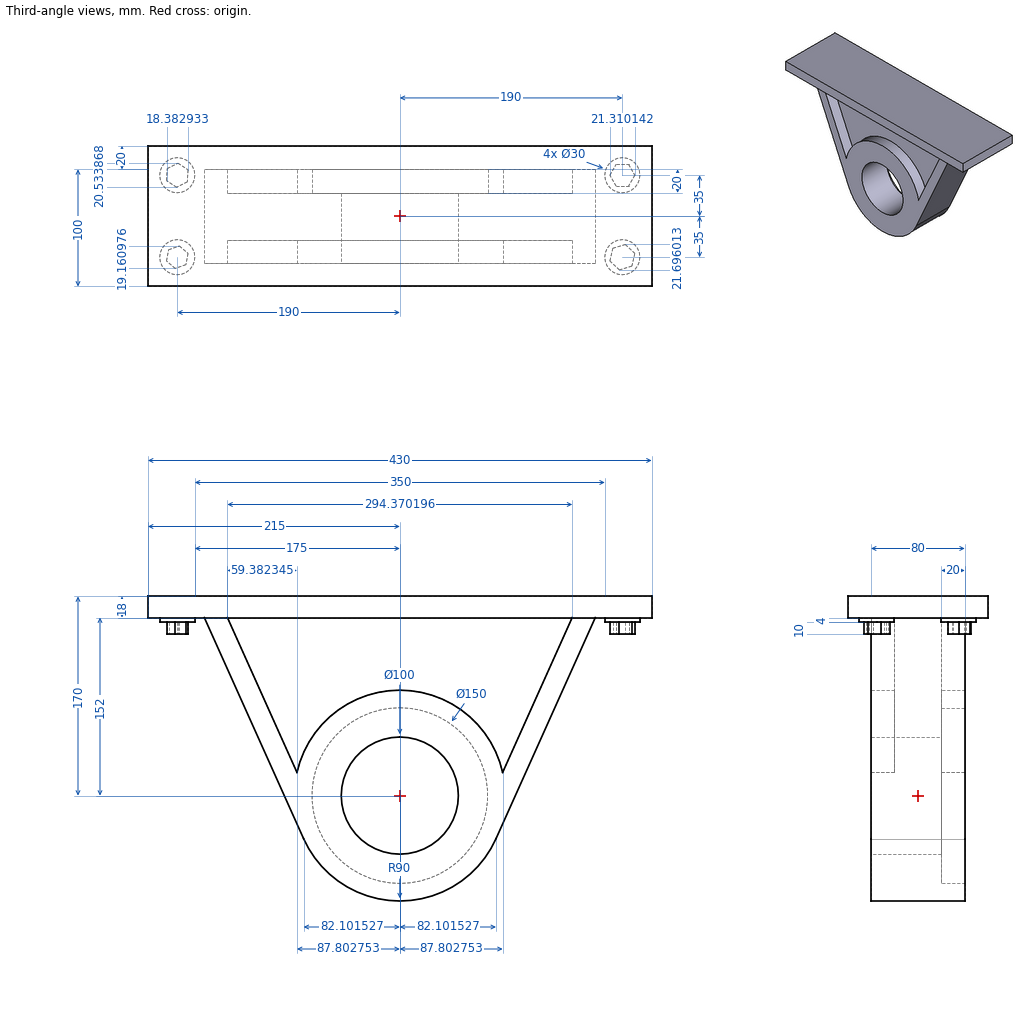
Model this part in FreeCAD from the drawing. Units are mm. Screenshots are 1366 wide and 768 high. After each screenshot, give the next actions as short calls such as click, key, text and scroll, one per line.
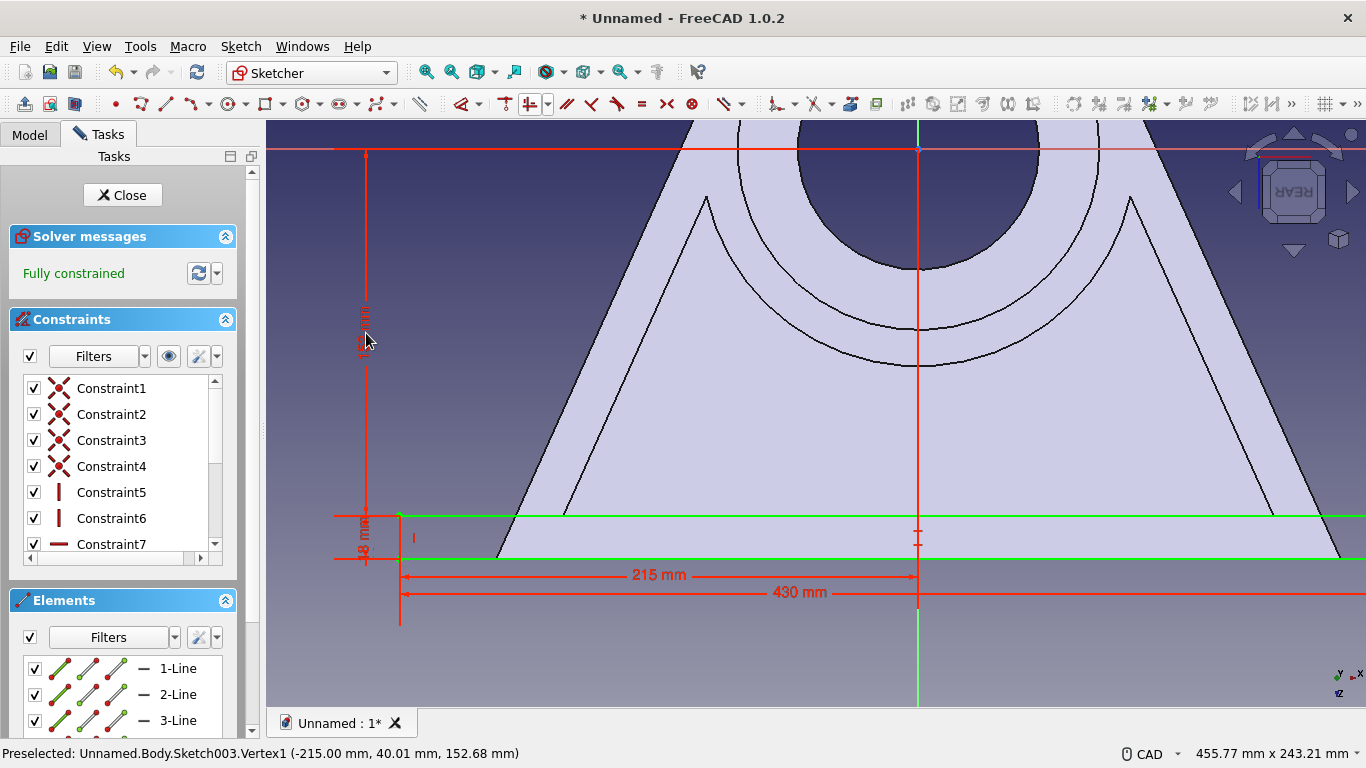
click(123, 195)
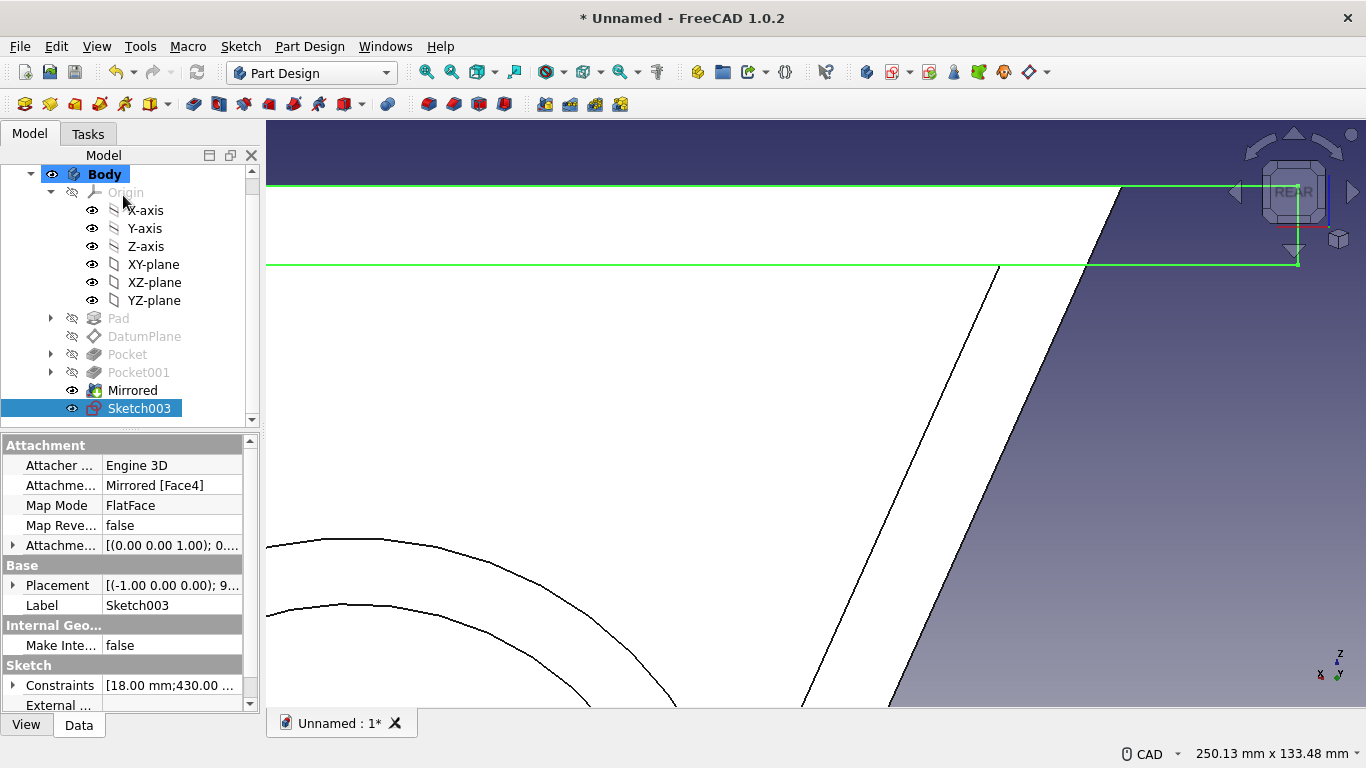
click(25, 104)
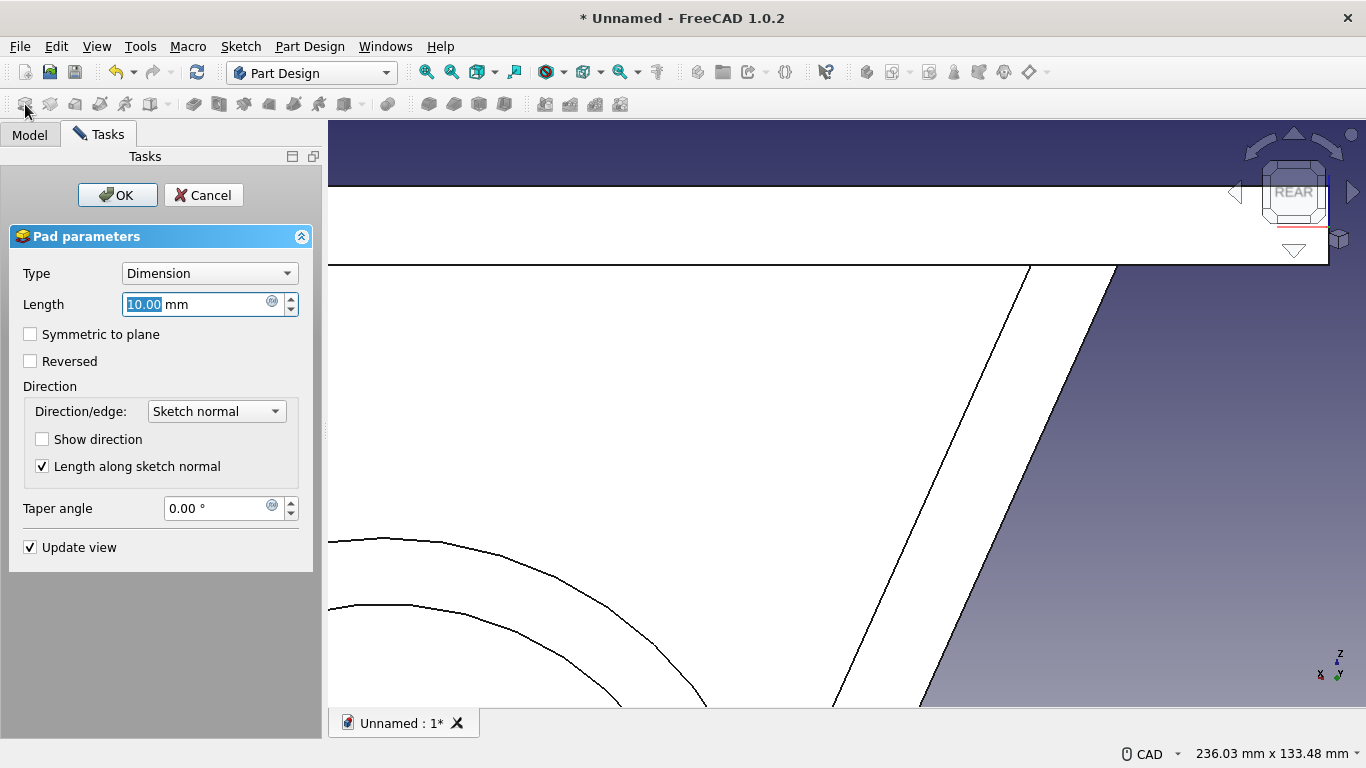
click(210, 274)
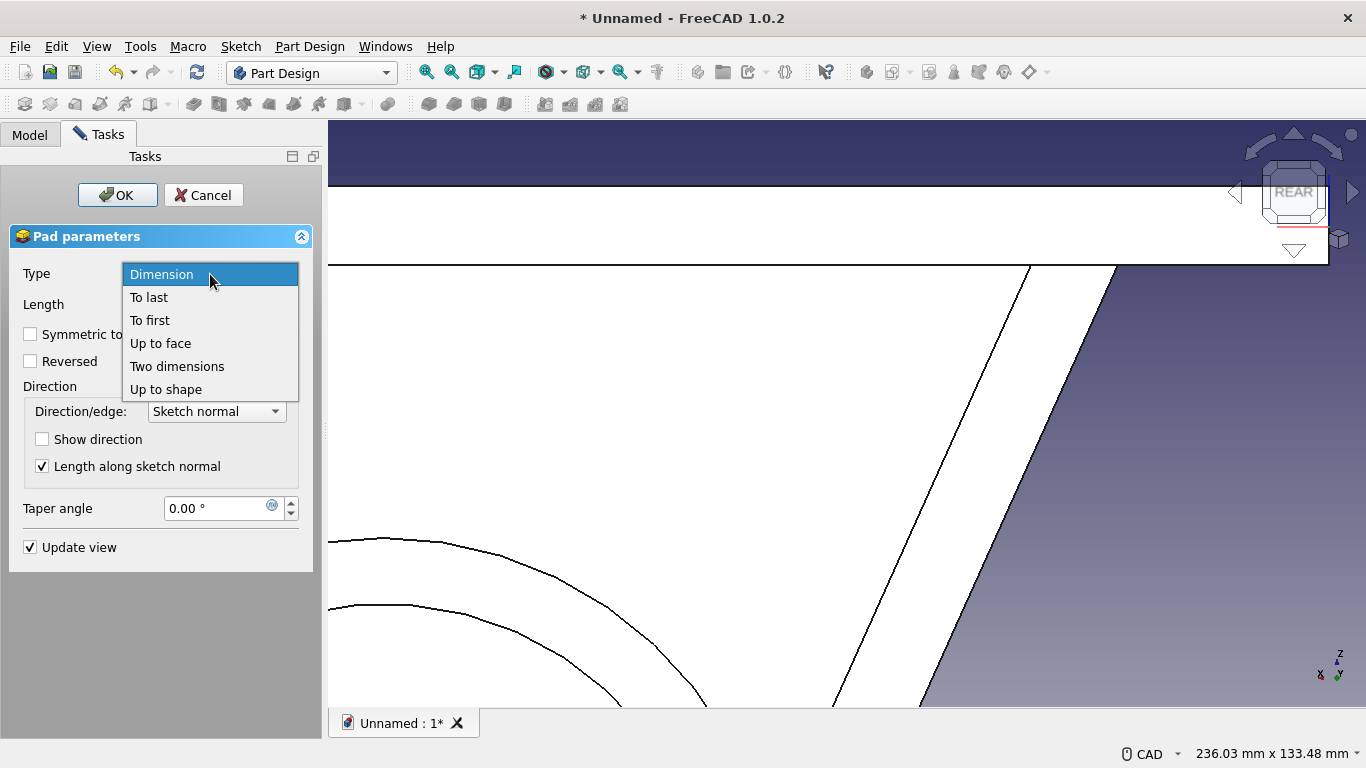
click(208, 366)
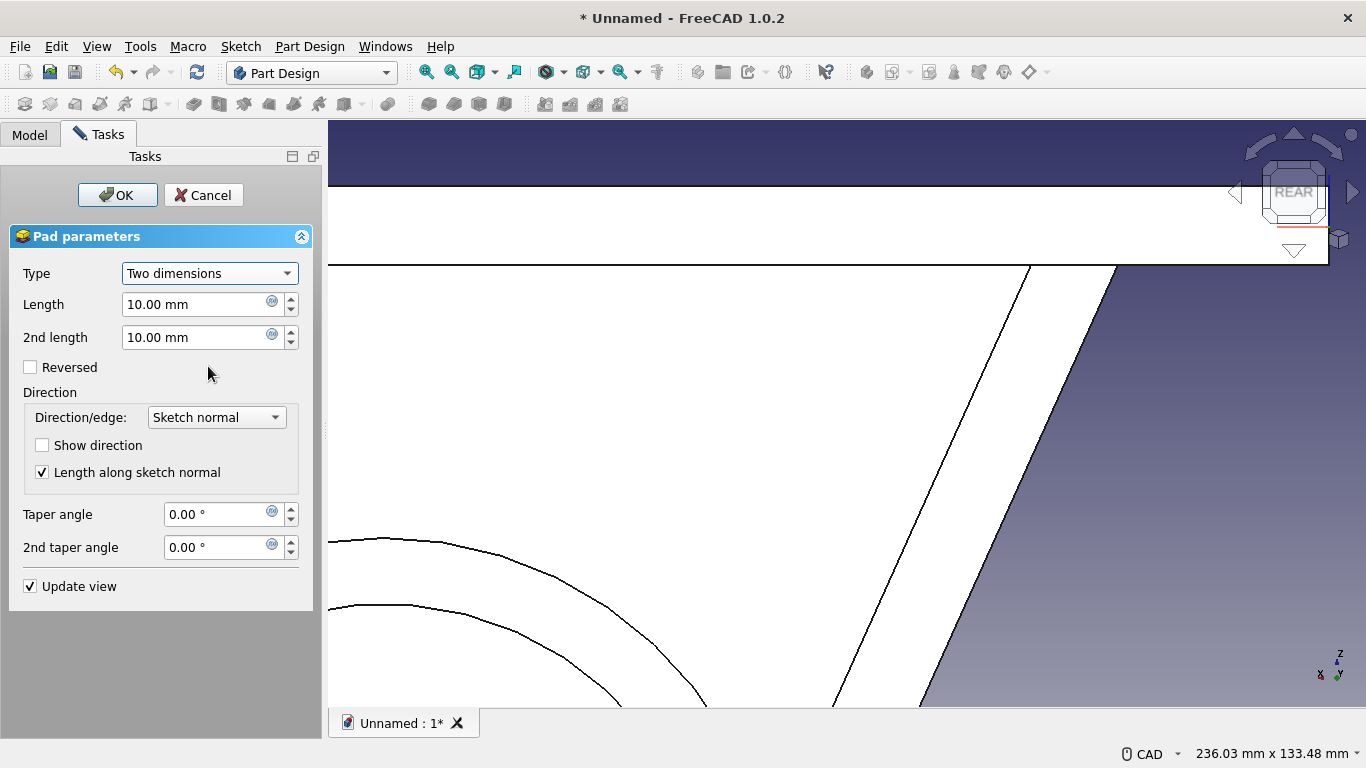
triple_click(204, 304)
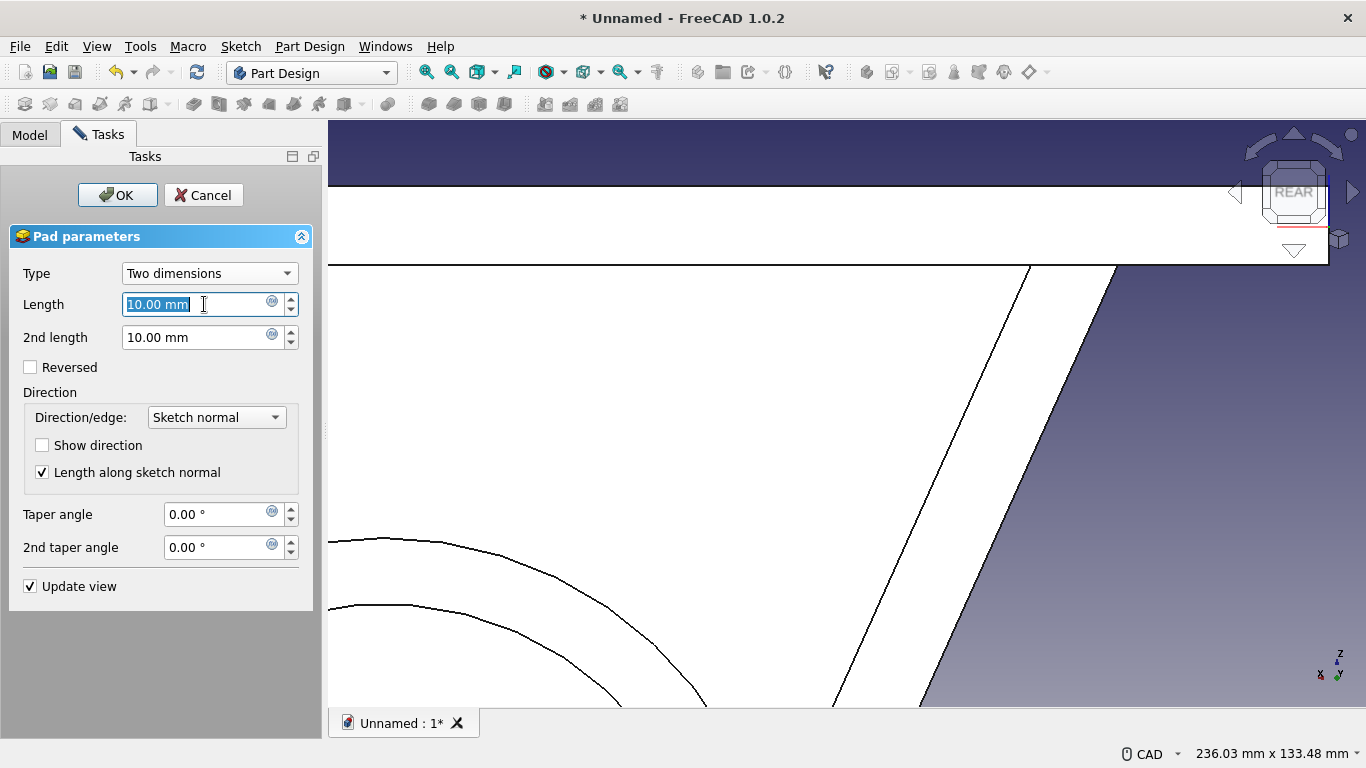
text(20)
key(Tab)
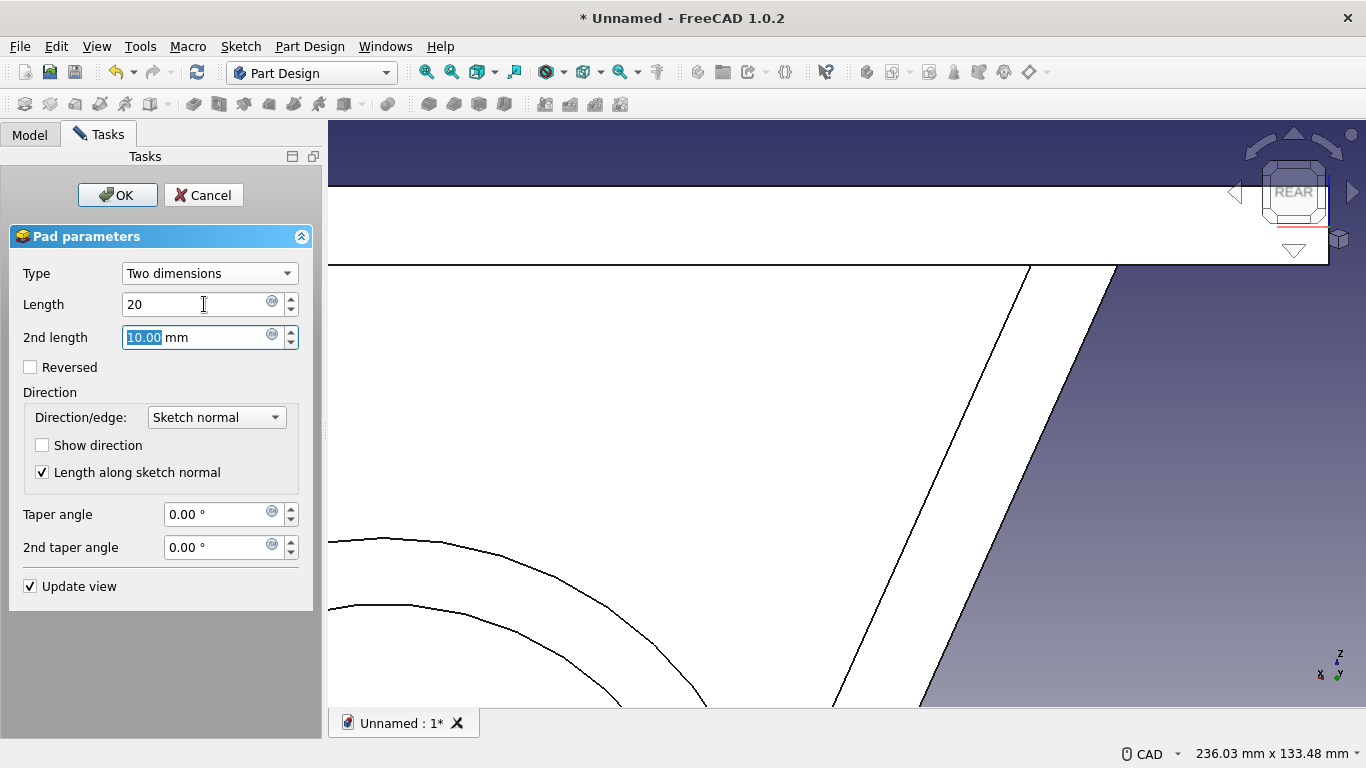
text(100)
key(Tab)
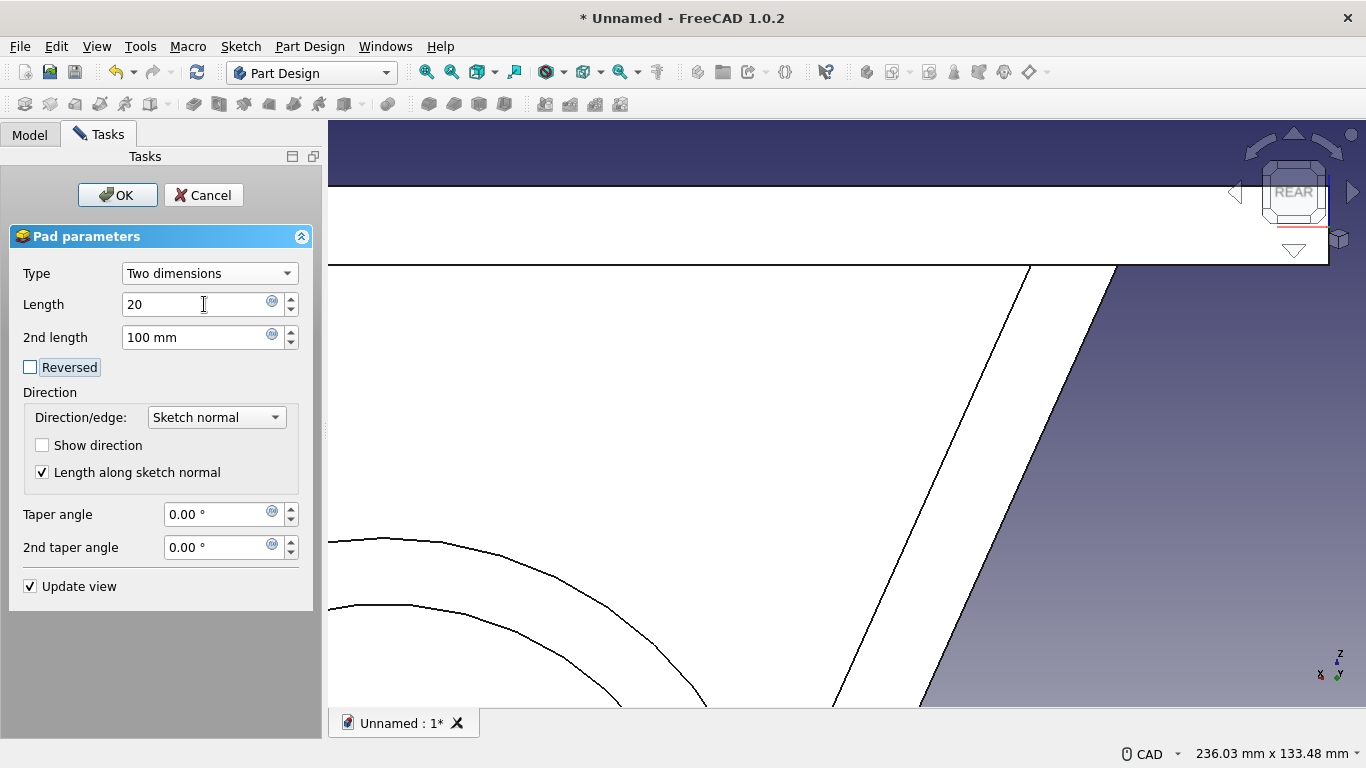
click(118, 195)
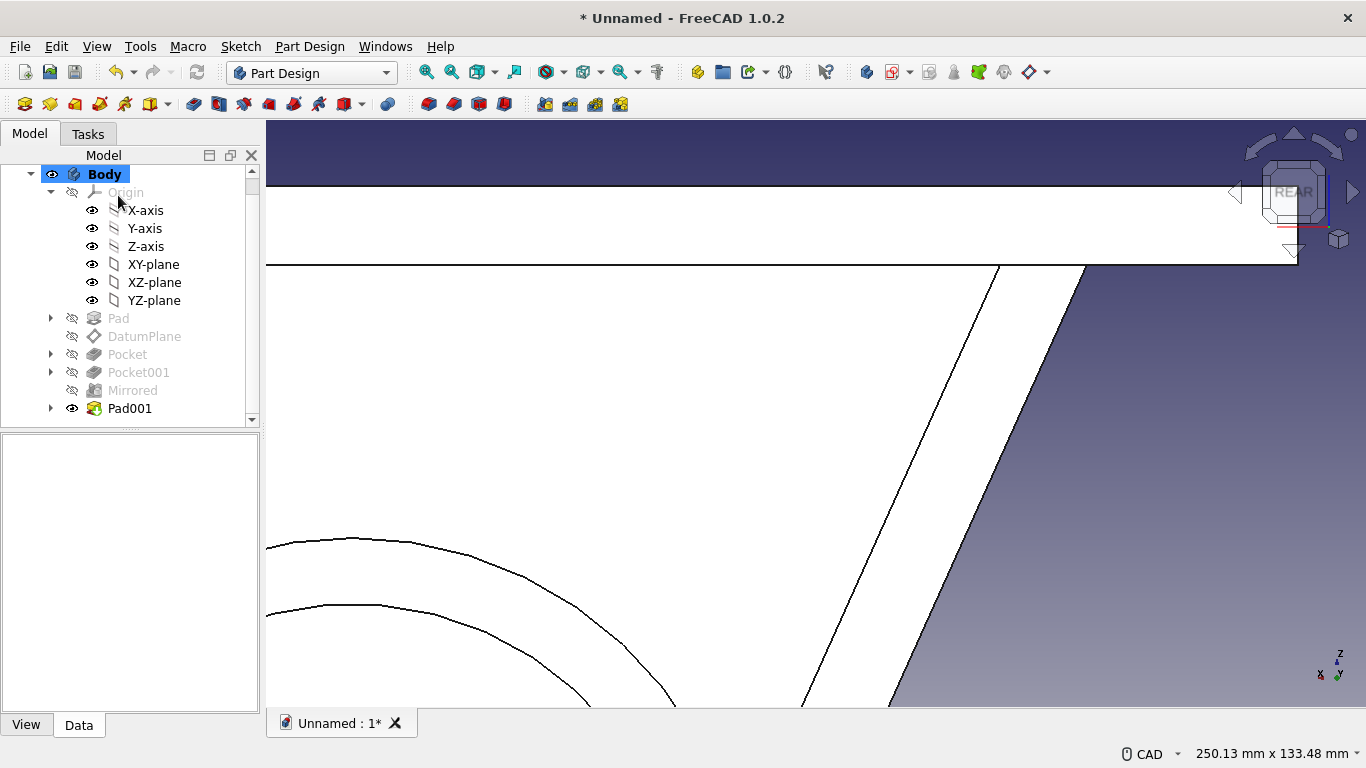
click(427, 72)